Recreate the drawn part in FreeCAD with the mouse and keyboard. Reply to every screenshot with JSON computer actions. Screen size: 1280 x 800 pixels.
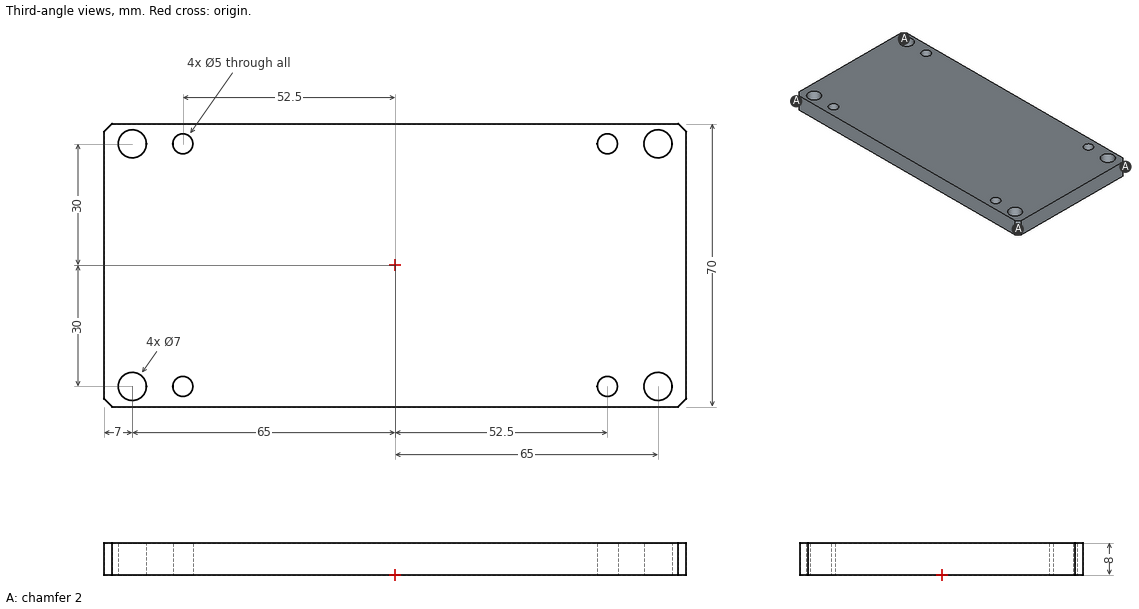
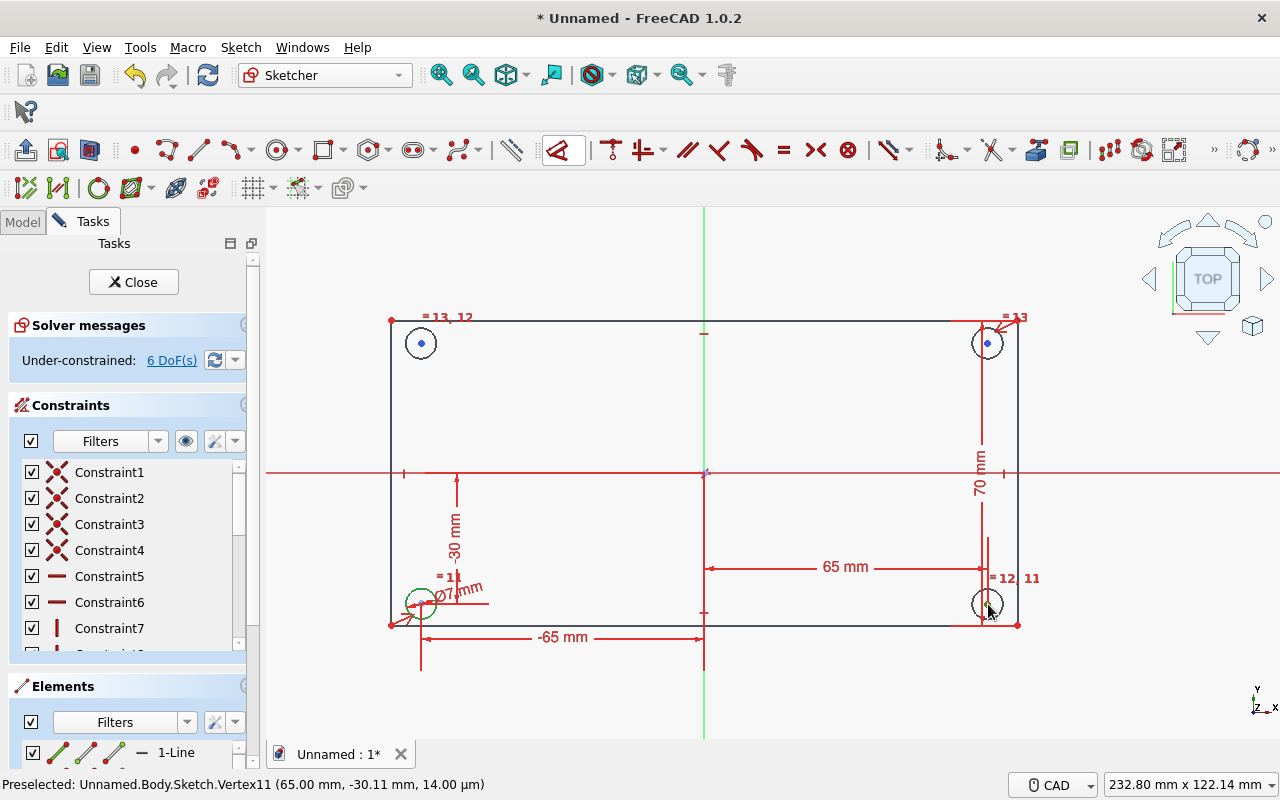
{"action": "key", "text": "i"}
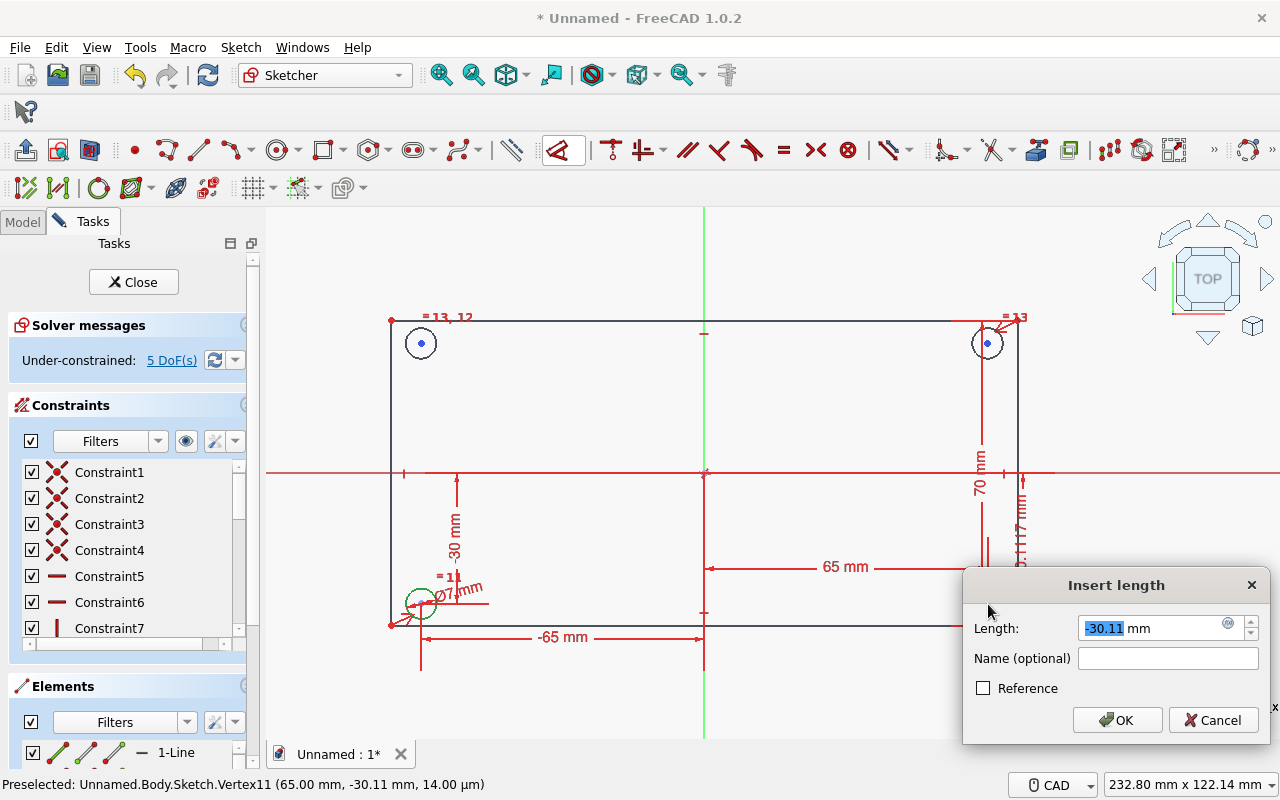
{"action": "type", "text": "-30"}
{"action": "key", "text": "Return"}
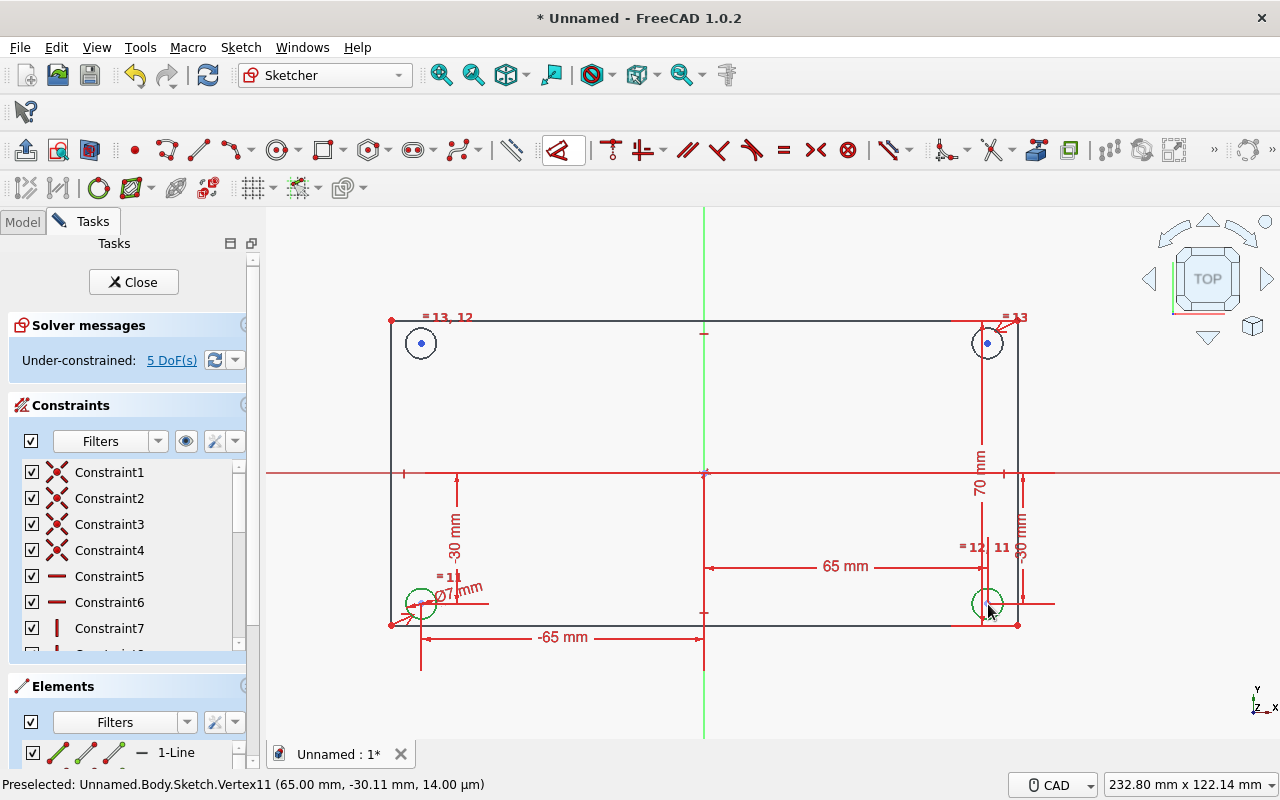
{"action": "left_click", "coordinate": [421, 343]}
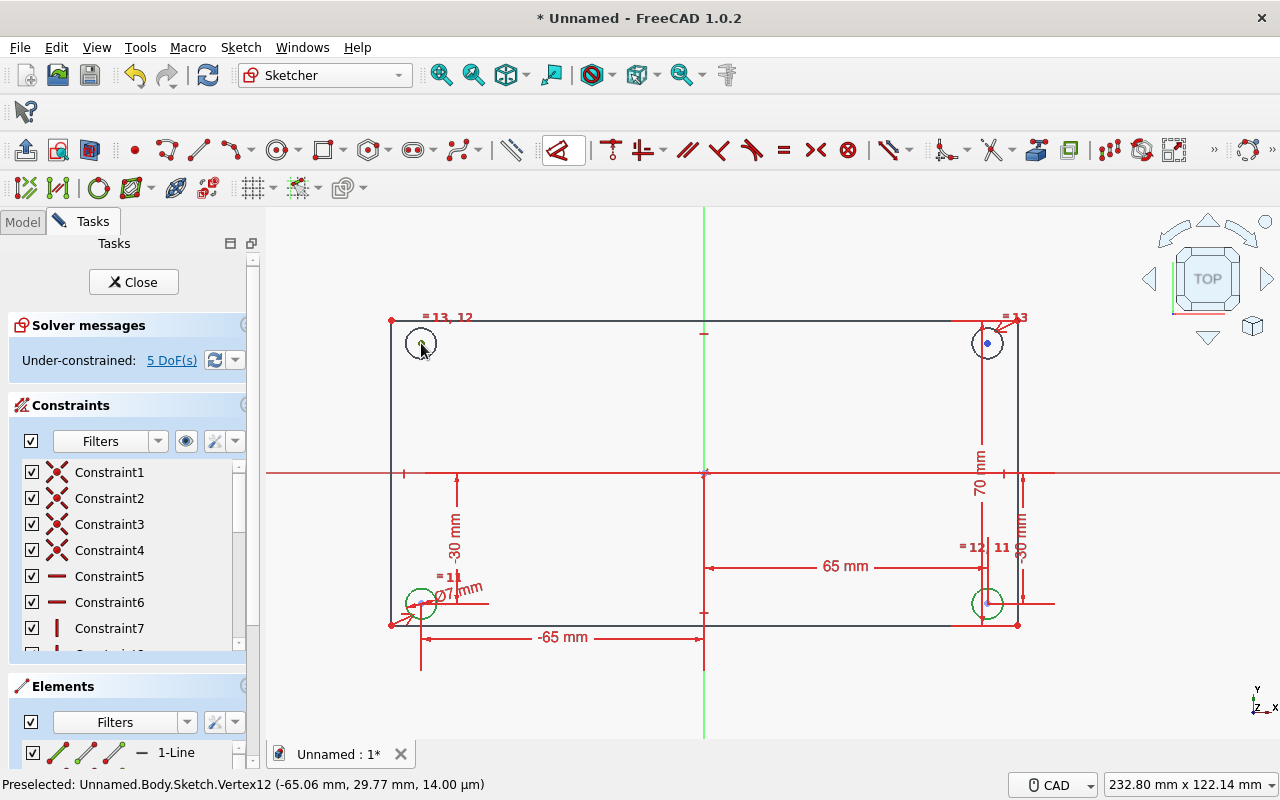
{"action": "key", "text": "l"}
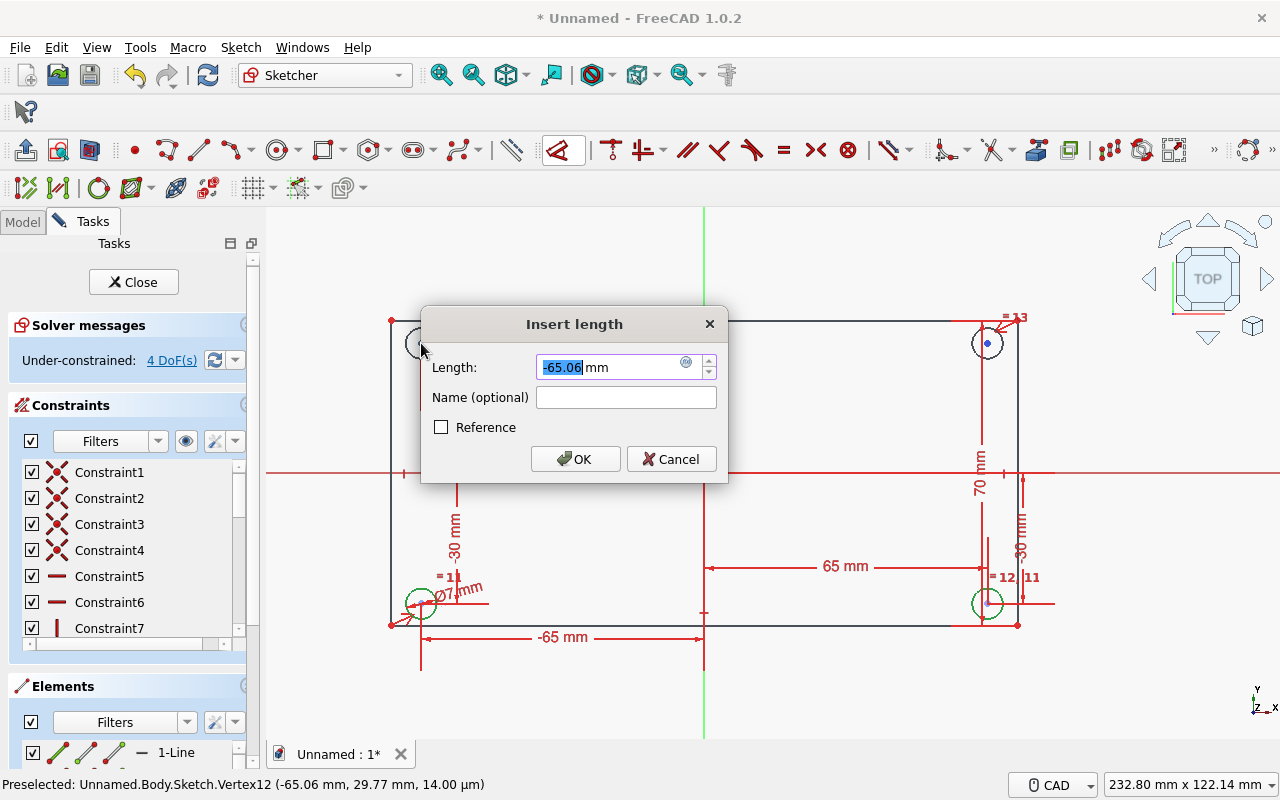
{"action": "type", "text": "-65"}
{"action": "key", "text": "Return"}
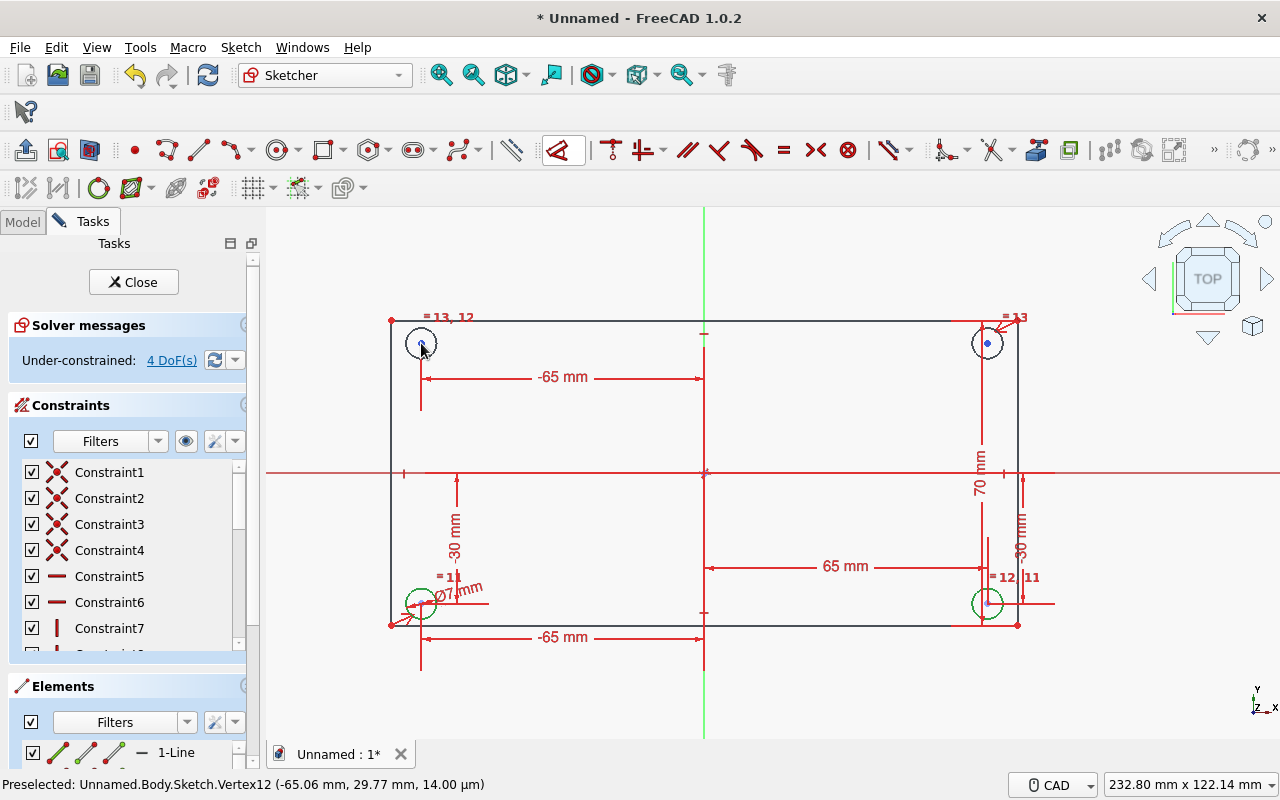
{"action": "left_click", "coordinate": [421, 343]}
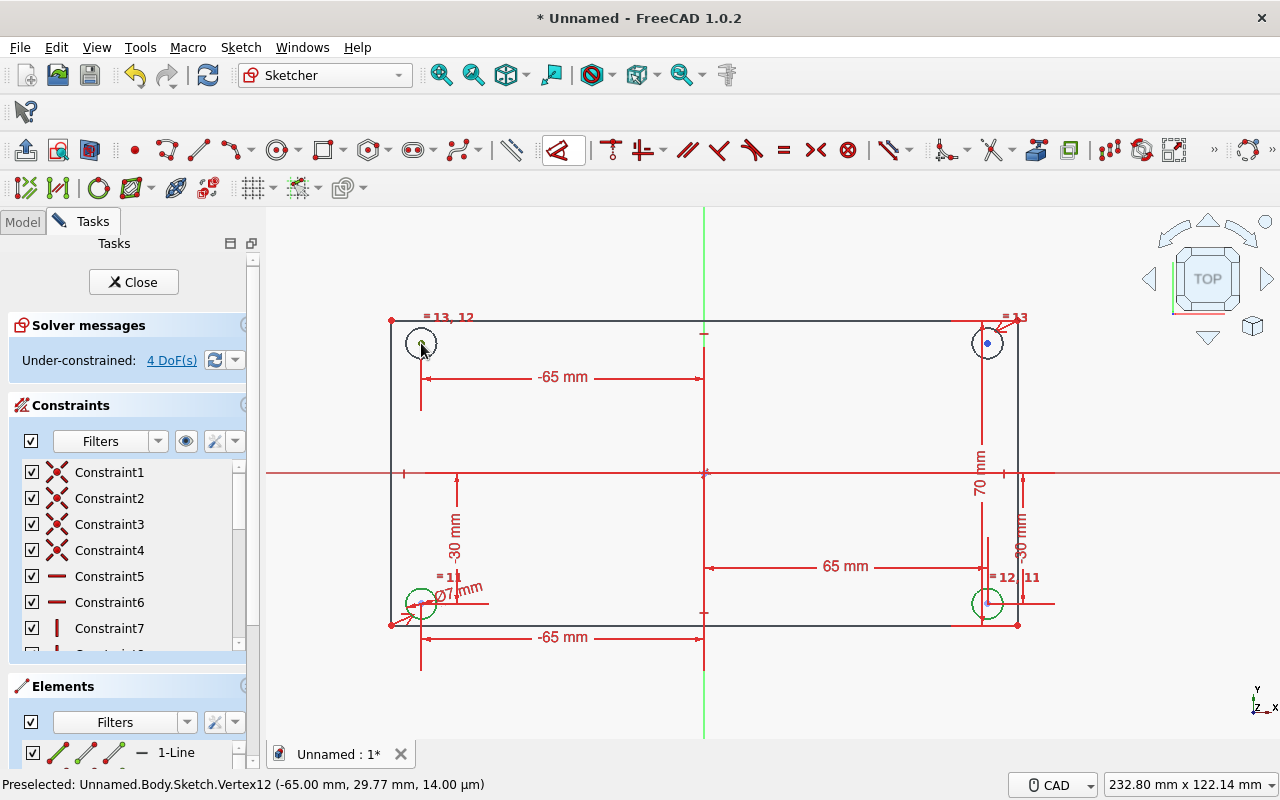
{"action": "key", "text": "i"}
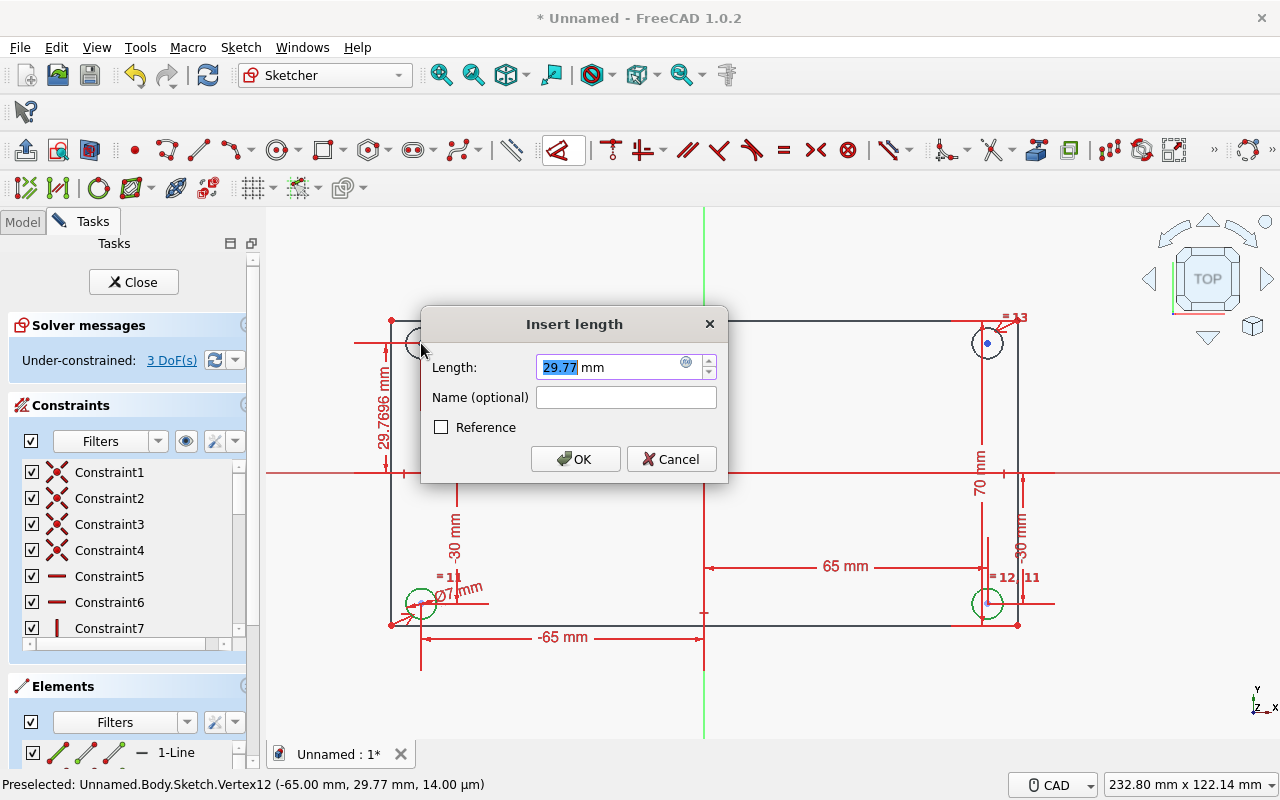
{"action": "type", "text": "30"}
{"action": "key", "text": "Return"}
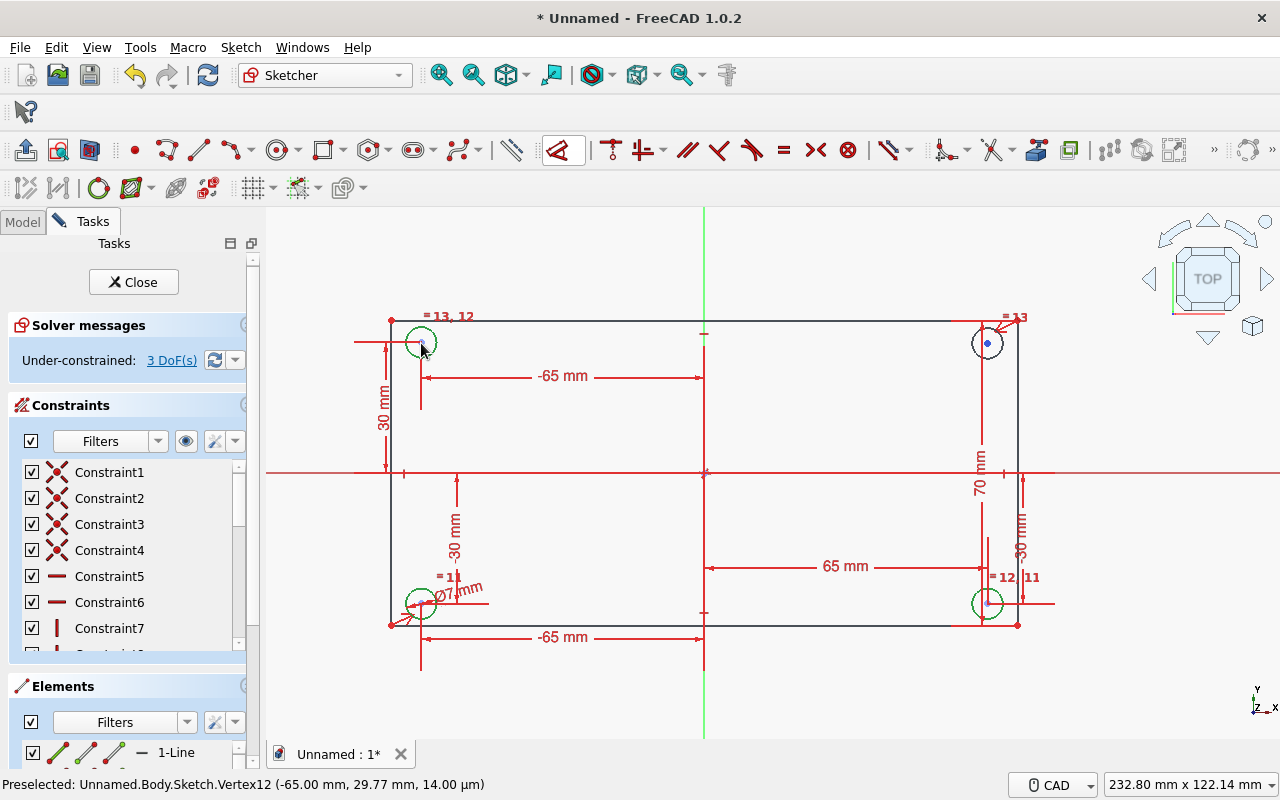
{"action": "left_click", "coordinate": [988, 343]}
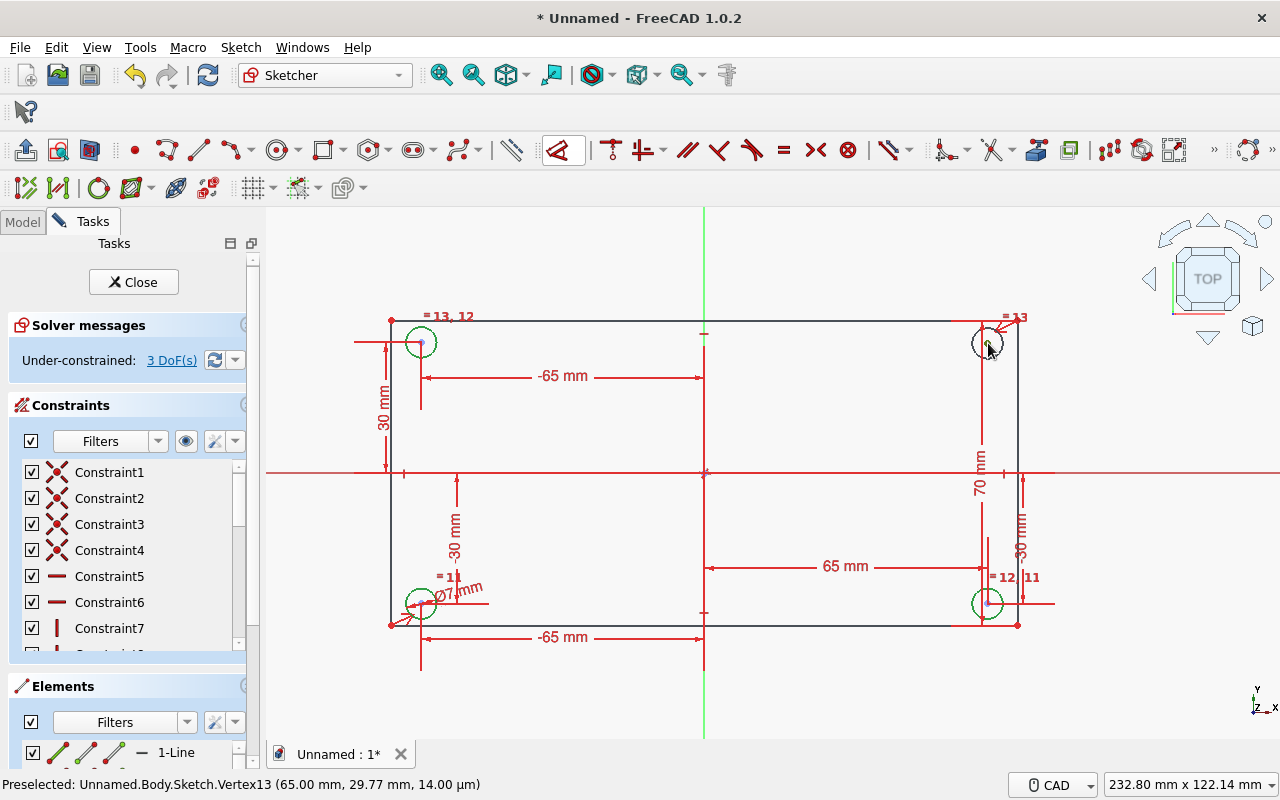
{"action": "left_click", "coordinate": [580, 150]}